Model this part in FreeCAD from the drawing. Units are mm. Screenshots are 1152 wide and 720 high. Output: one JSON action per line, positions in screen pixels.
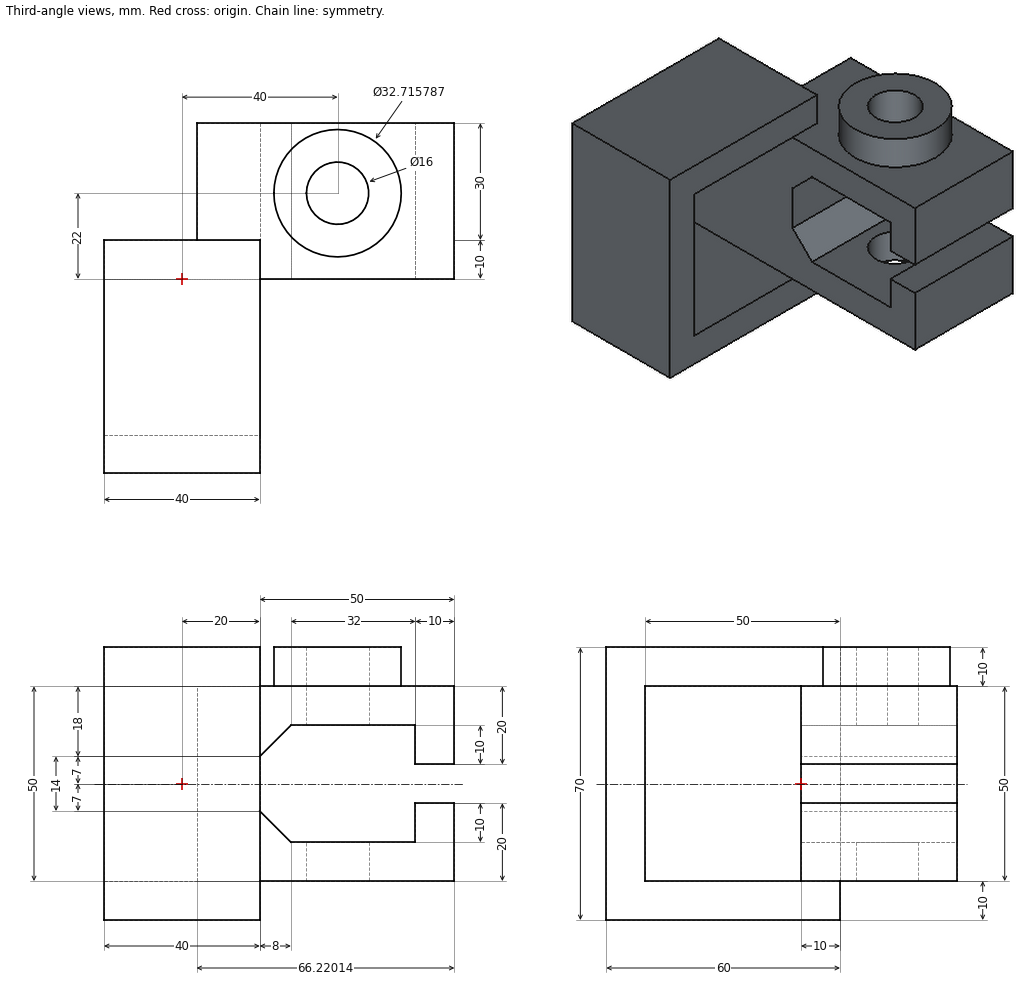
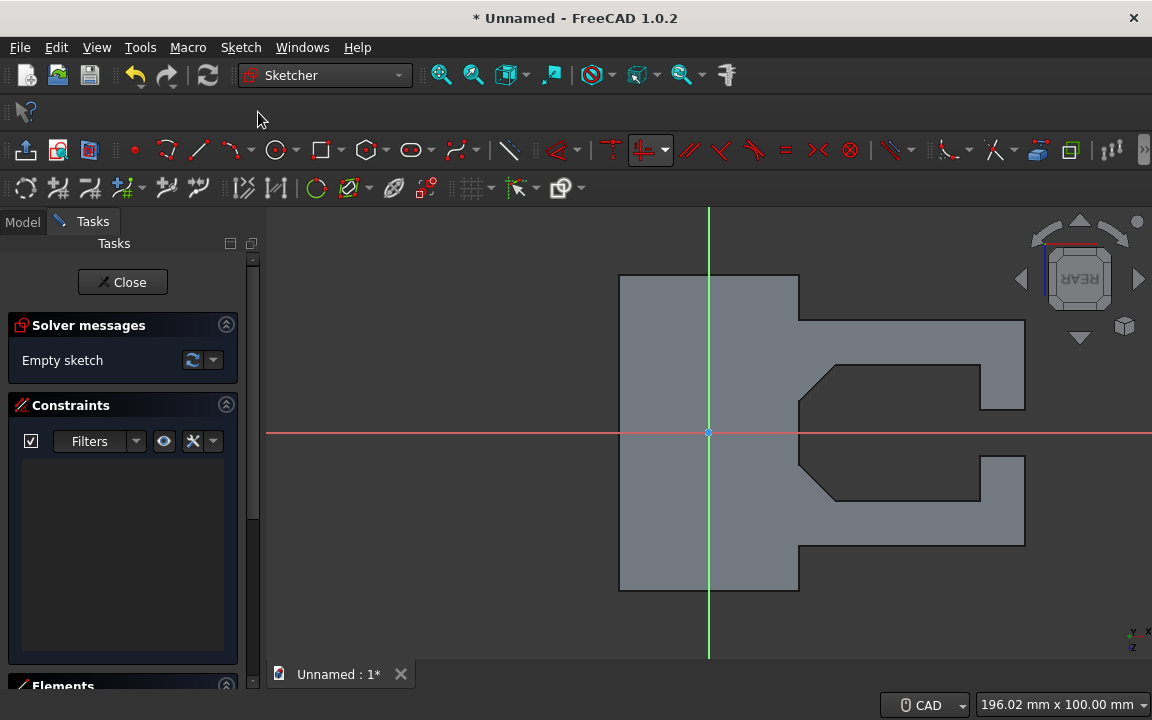
{"action": "scroll", "coordinate": [294, 433], "scroll_direction": "down", "scroll_amount": 1}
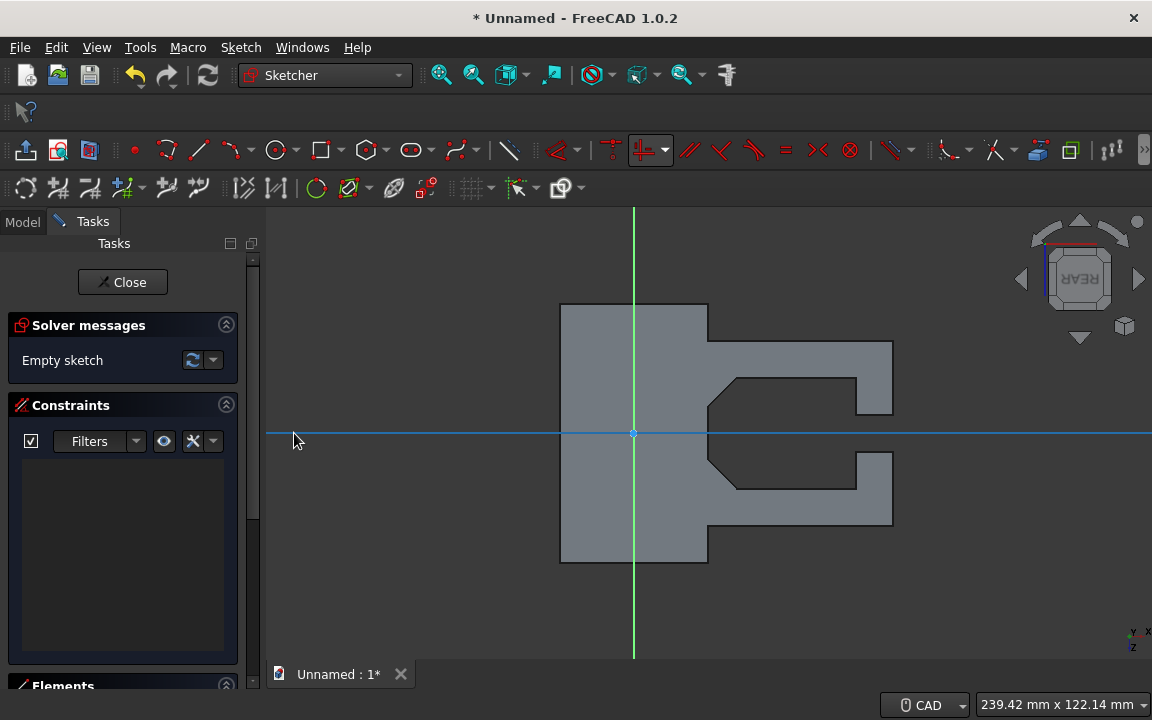
{"action": "scroll", "coordinate": [987, 433], "scroll_direction": "up", "scroll_amount": 2}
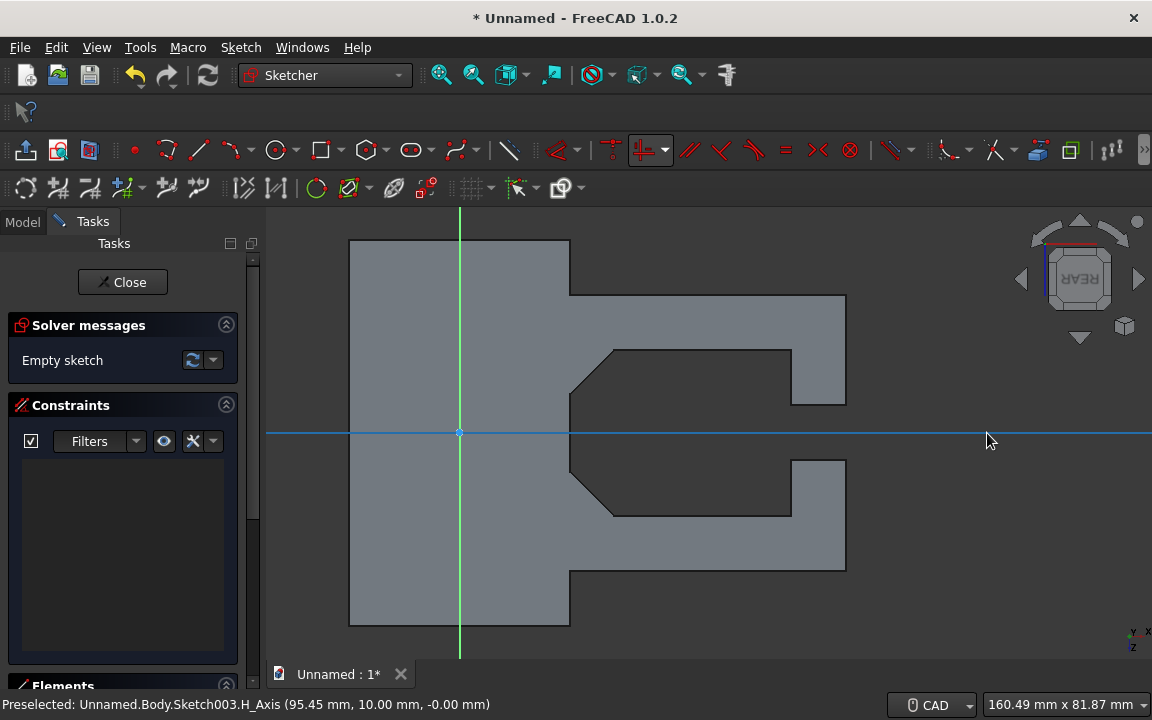
{"action": "left_click", "coordinate": [168, 150]}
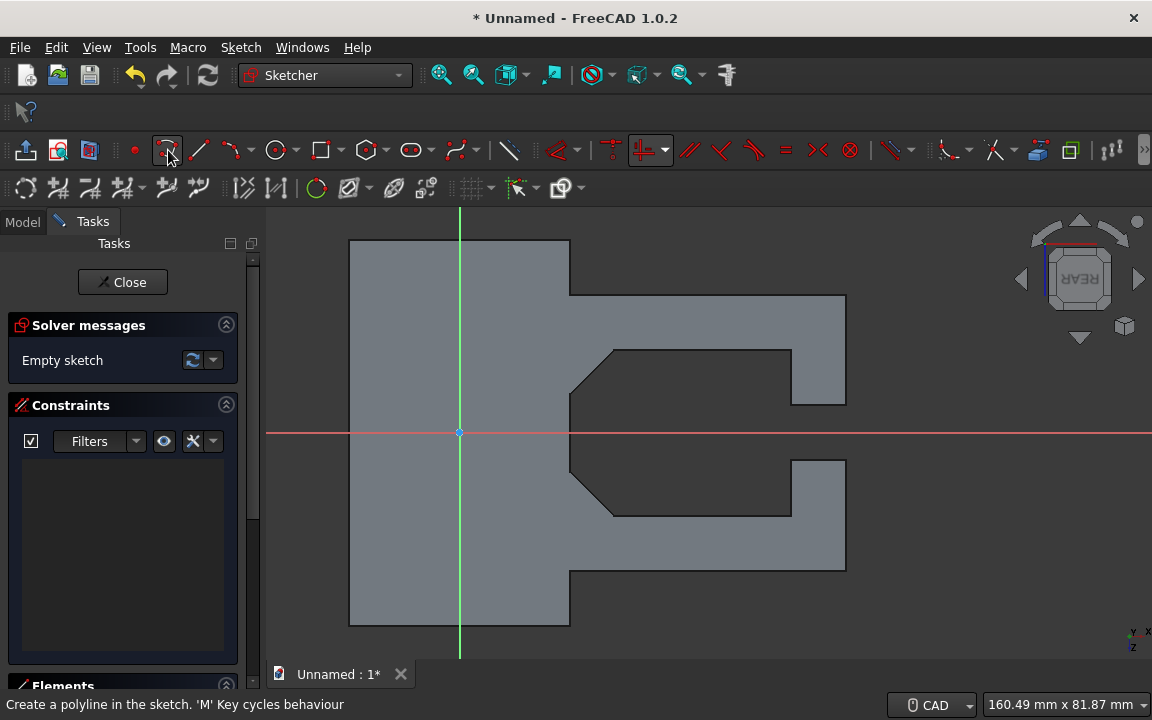
{"action": "left_click", "coordinate": [570, 394]}
{"action": "left_click", "coordinate": [614, 350]}
{"action": "left_click", "coordinate": [791, 350]}
{"action": "left_click", "coordinate": [791, 405]}
{"action": "left_click", "coordinate": [846, 405]}
{"action": "left_click", "coordinate": [846, 295]}
{"action": "left_click", "coordinate": [481, 295]}
{"action": "left_click", "coordinate": [481, 571]}
{"action": "left_click", "coordinate": [846, 571]}
{"action": "left_click", "coordinate": [846, 460]}
{"action": "left_click", "coordinate": [791, 460]}
{"action": "left_click", "coordinate": [791, 516]}
{"action": "left_click", "coordinate": [614, 516]}
{"action": "left_click", "coordinate": [570, 472]}
{"action": "left_click", "coordinate": [570, 395]}
{"action": "key", "text": "Escape"}
{"action": "key", "text": "Escape"}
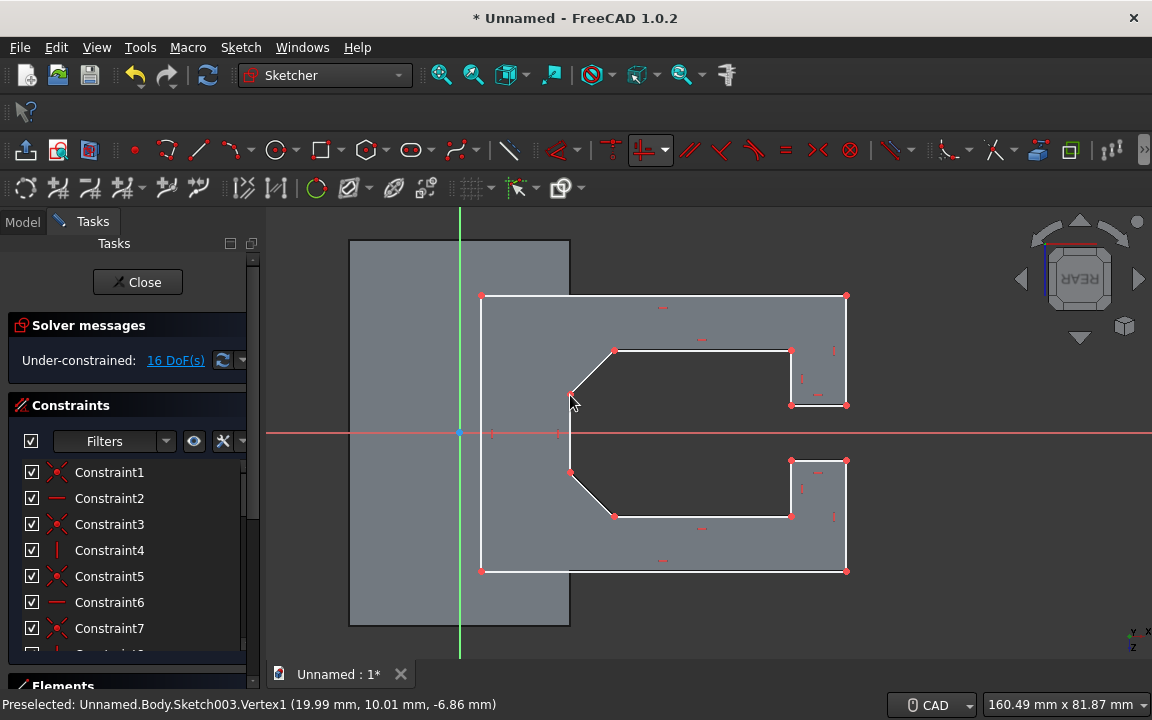
{"action": "left_click", "coordinate": [846, 296]}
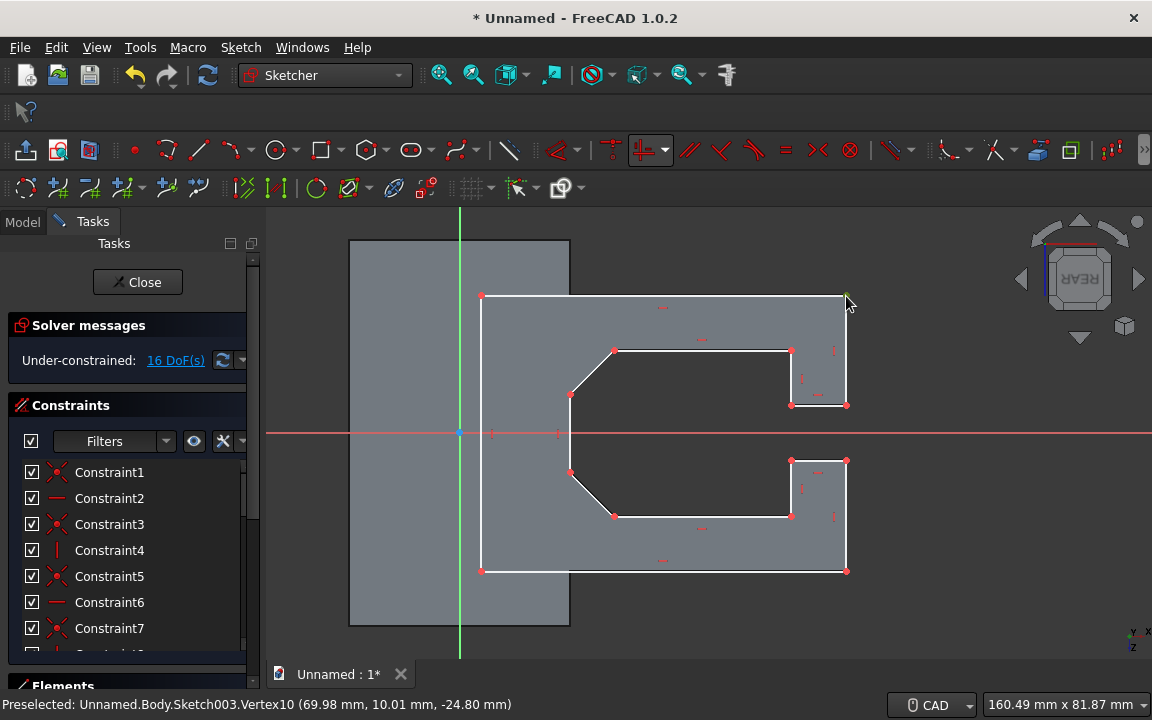
{"action": "left_click", "coordinate": [846, 572]}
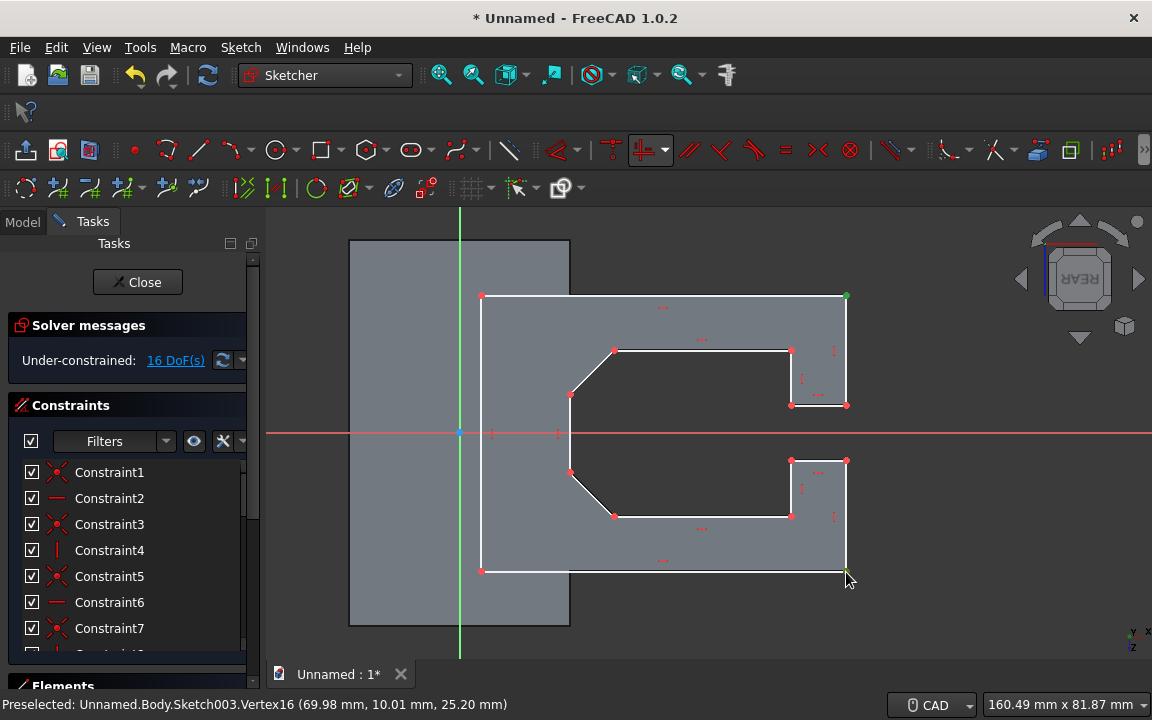
{"action": "left_click", "coordinate": [344, 433]}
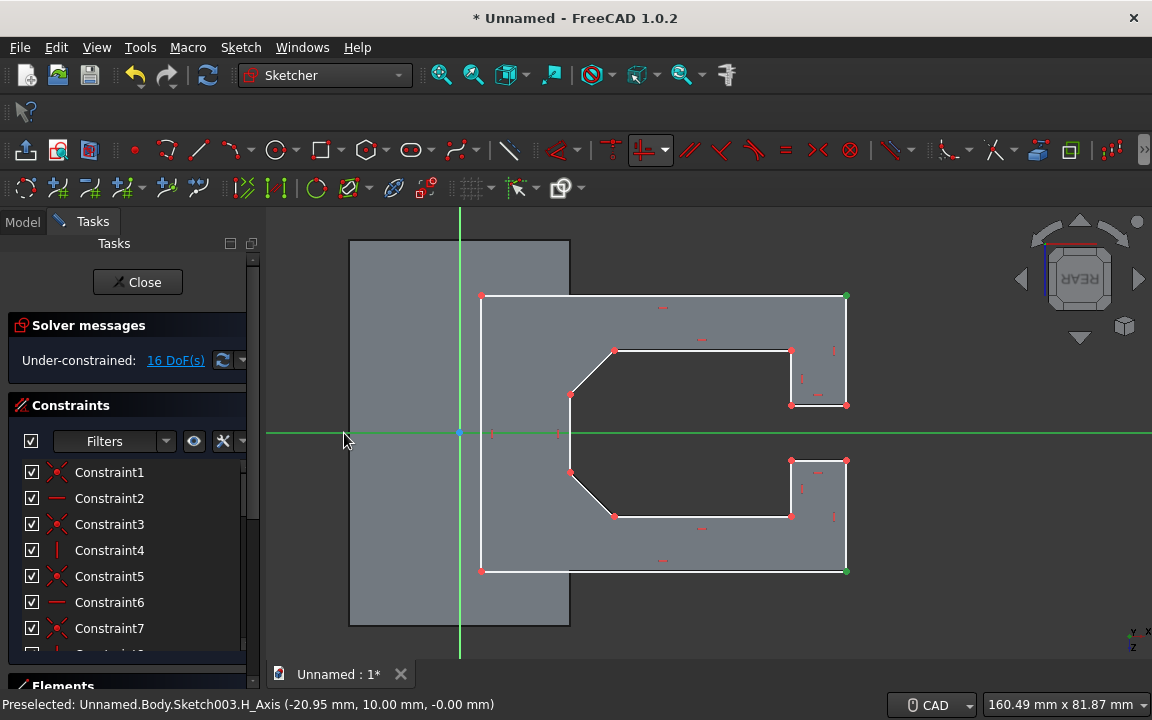
{"action": "key", "text": "s"}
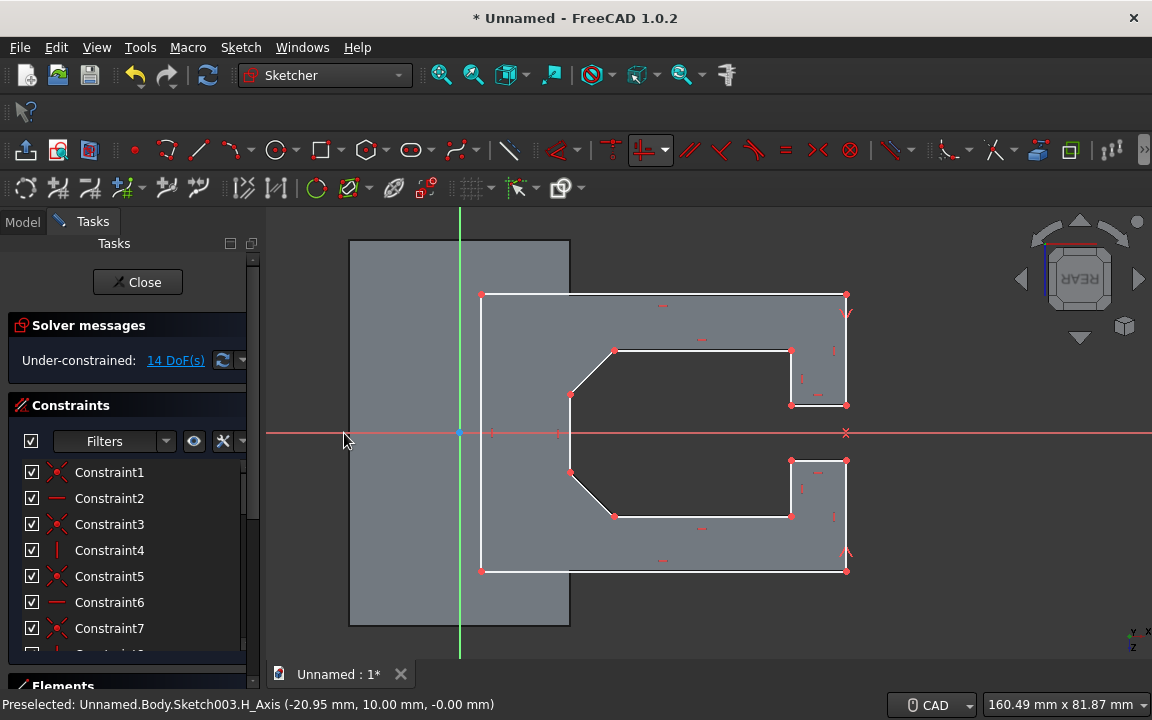
{"action": "left_click", "coordinate": [791, 406]}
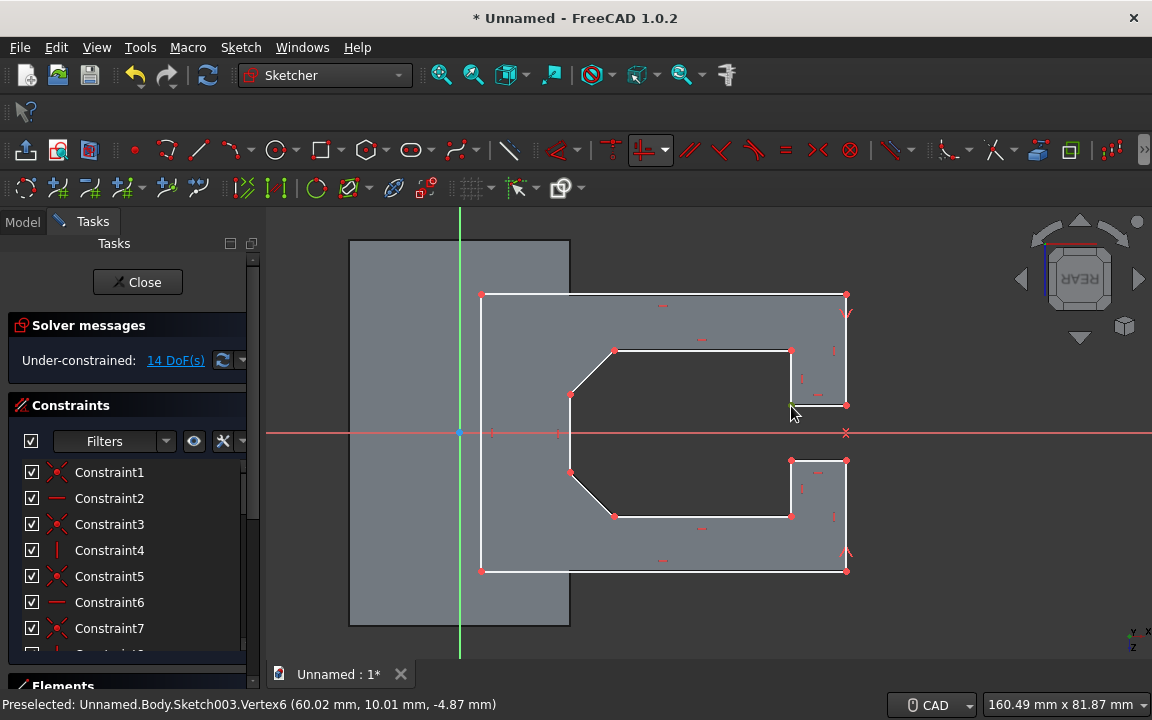
{"action": "left_click", "coordinate": [791, 461]}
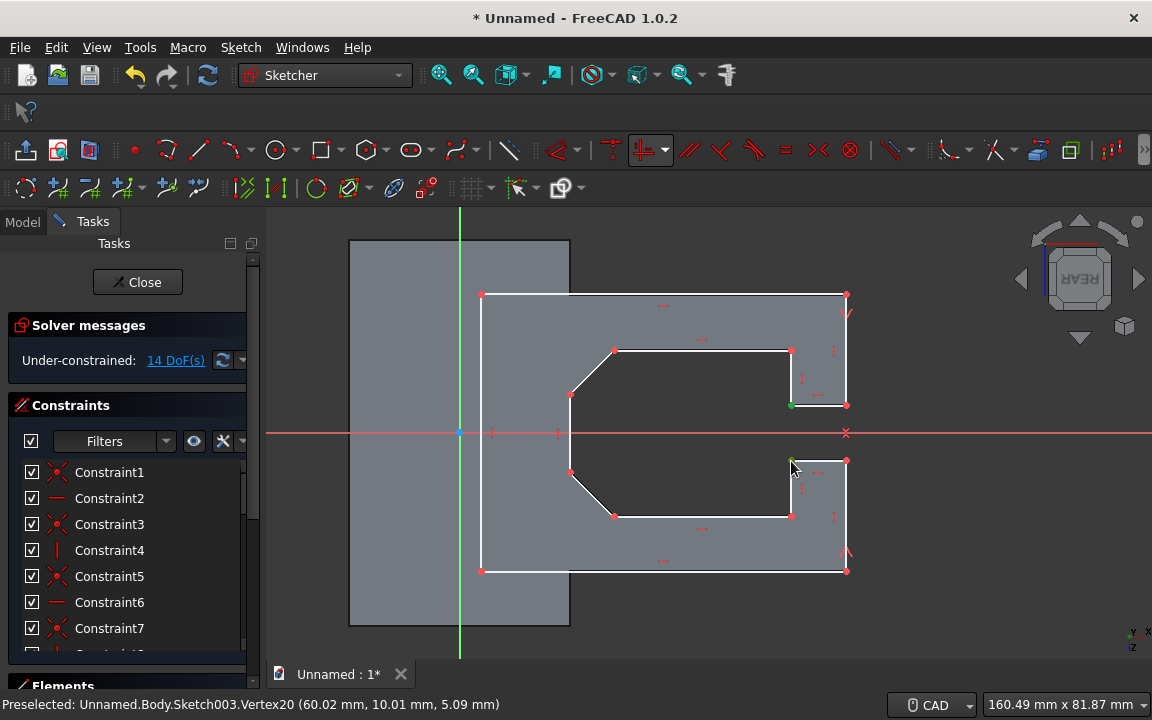
{"action": "left_click", "coordinate": [344, 433]}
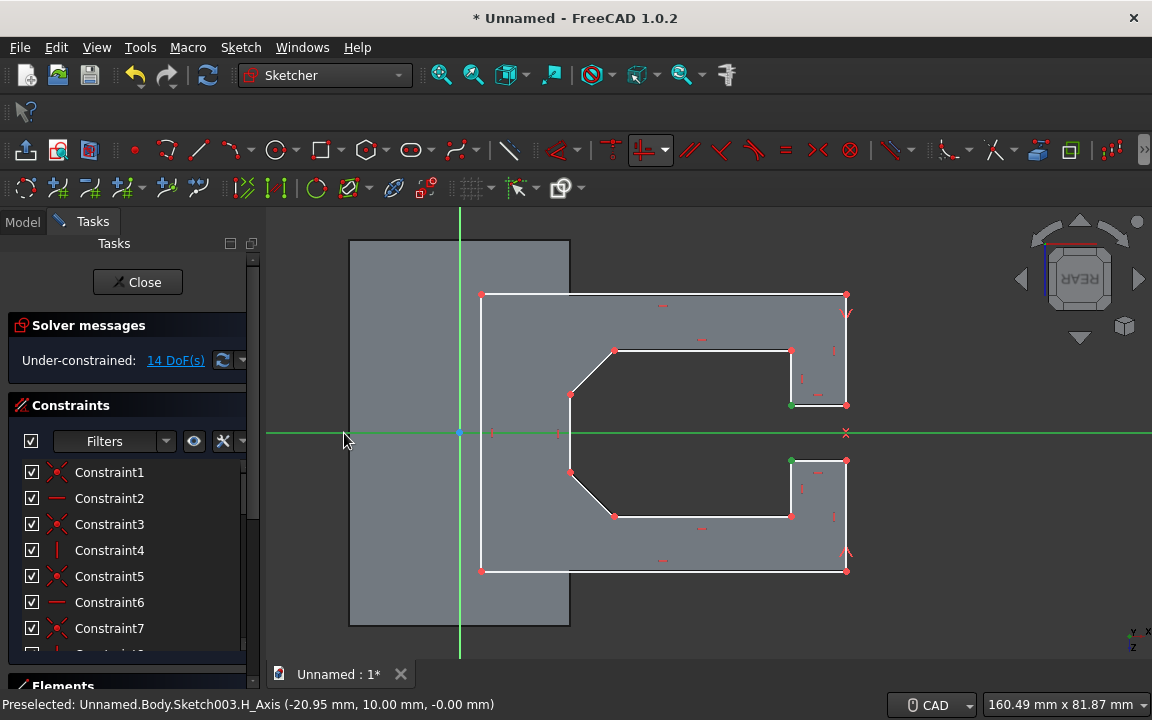
{"action": "key", "text": "s"}